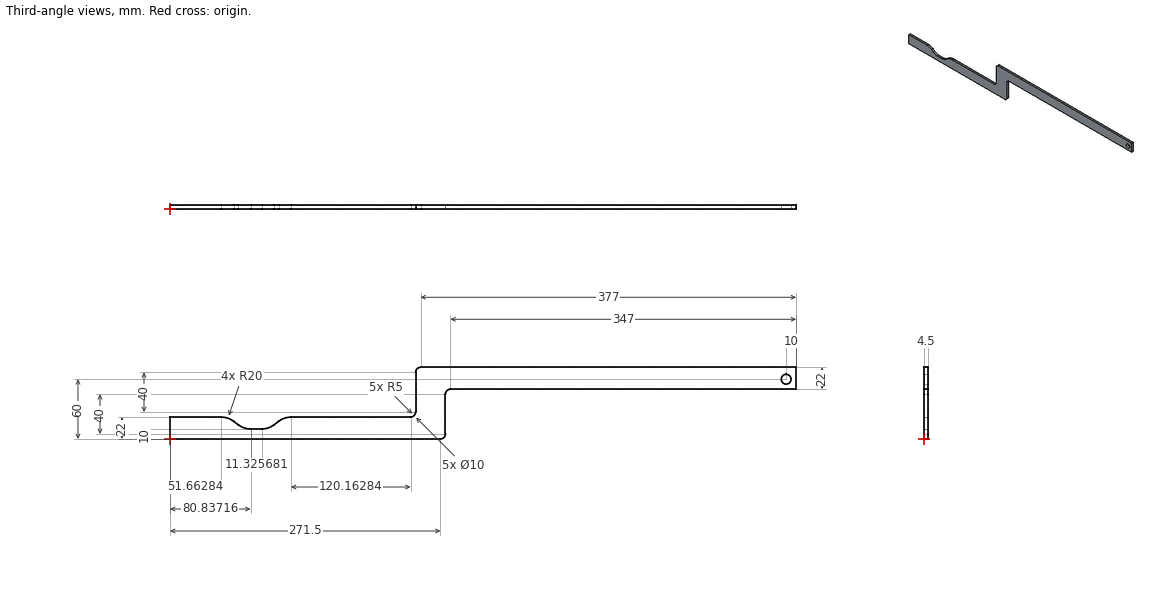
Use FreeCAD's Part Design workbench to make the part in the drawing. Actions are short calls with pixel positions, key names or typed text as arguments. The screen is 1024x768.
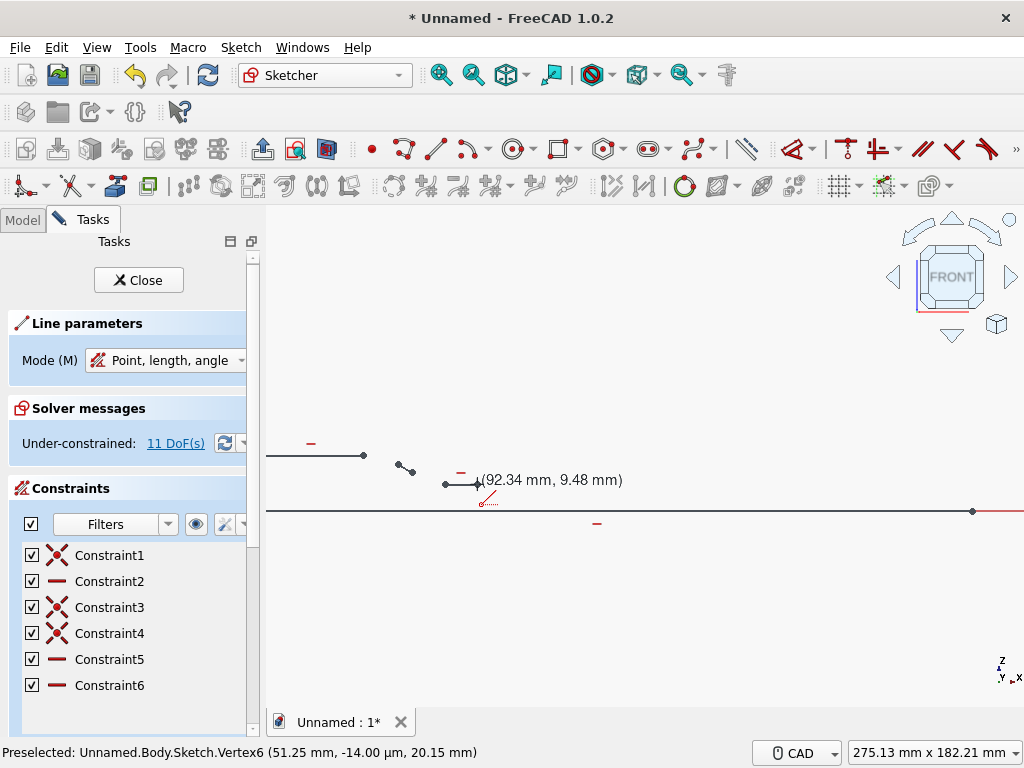
click(510, 472)
click(523, 462)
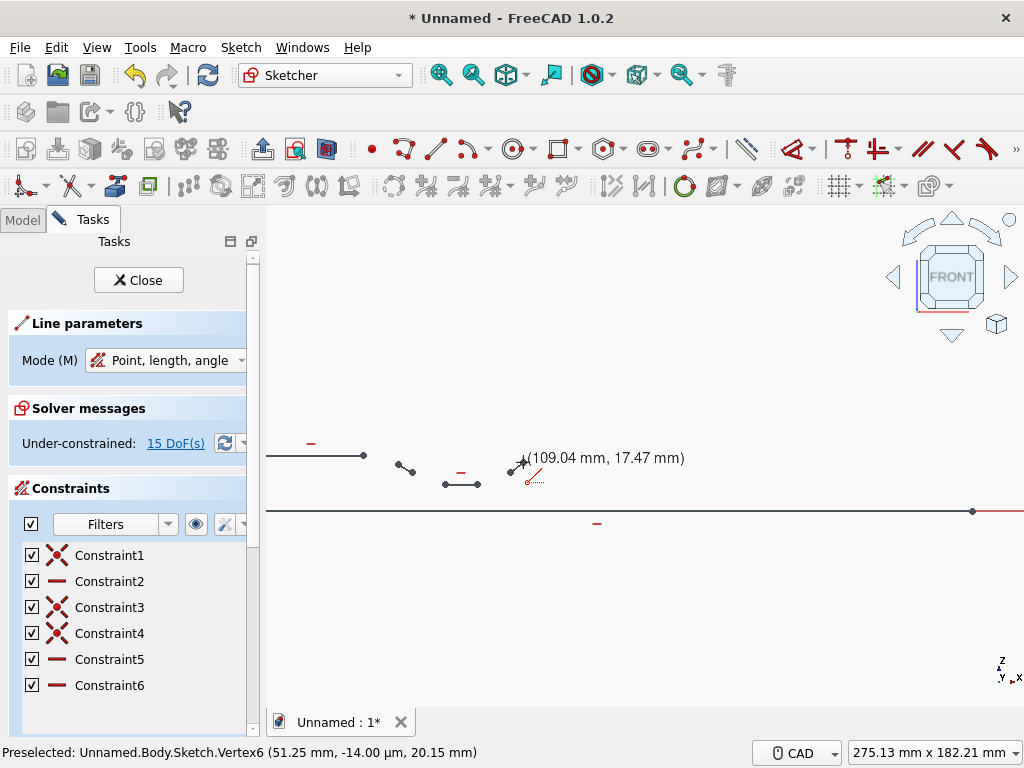
click(557, 451)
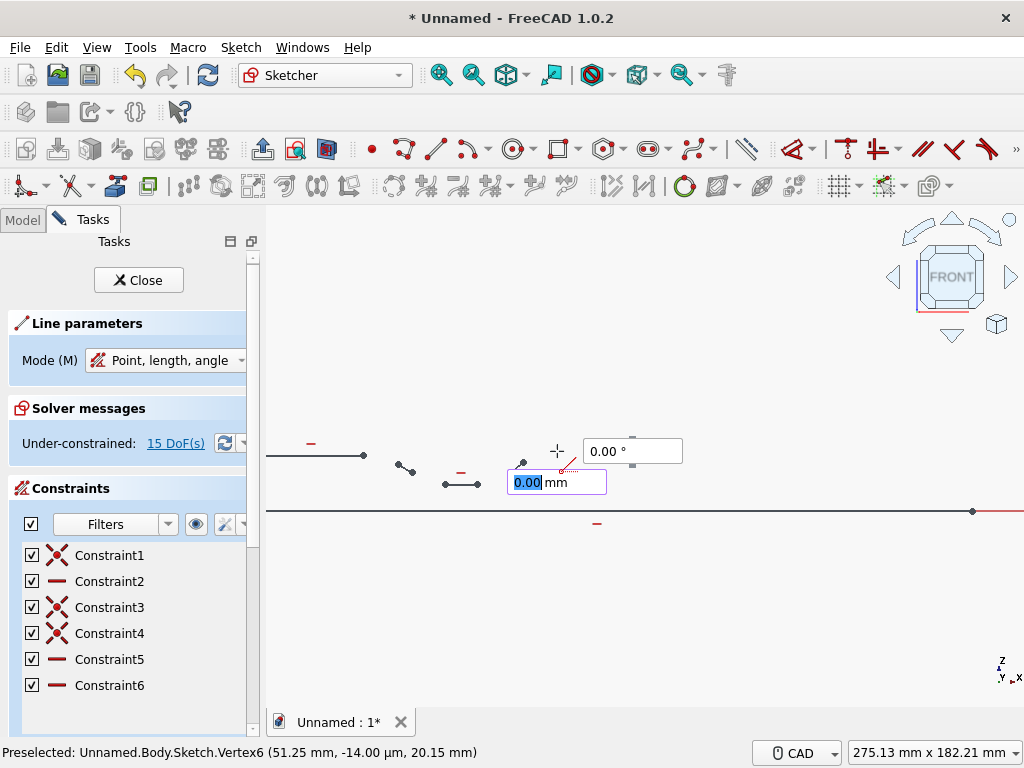
scroll(409, 470, down, 7)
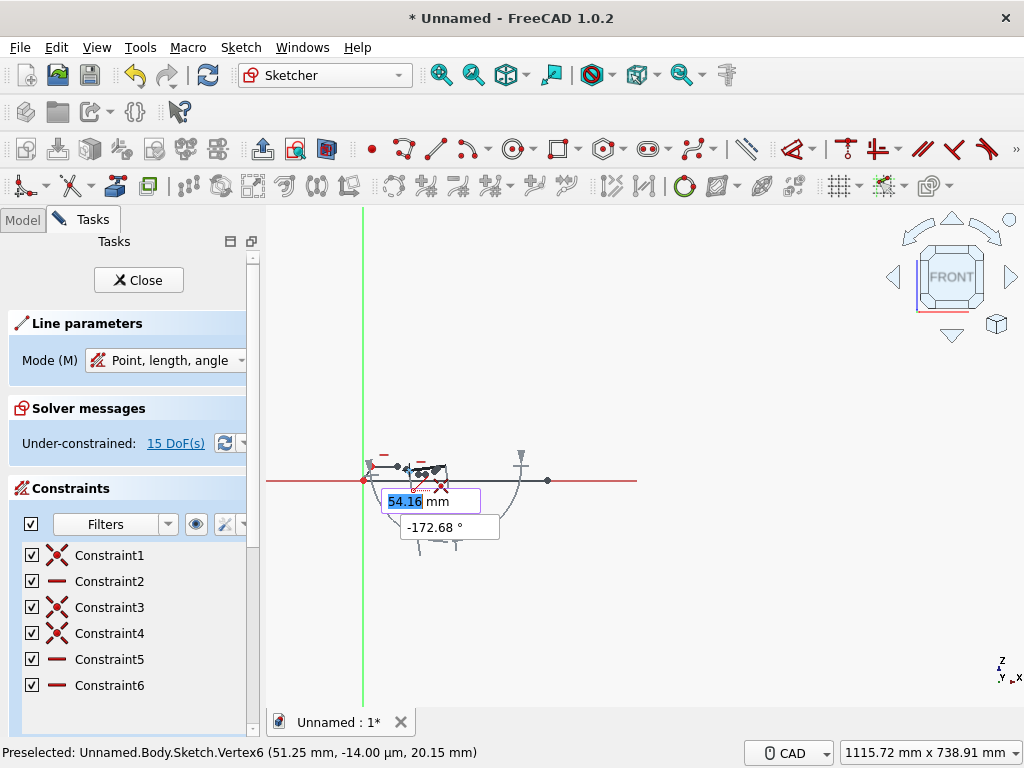
click(527, 466)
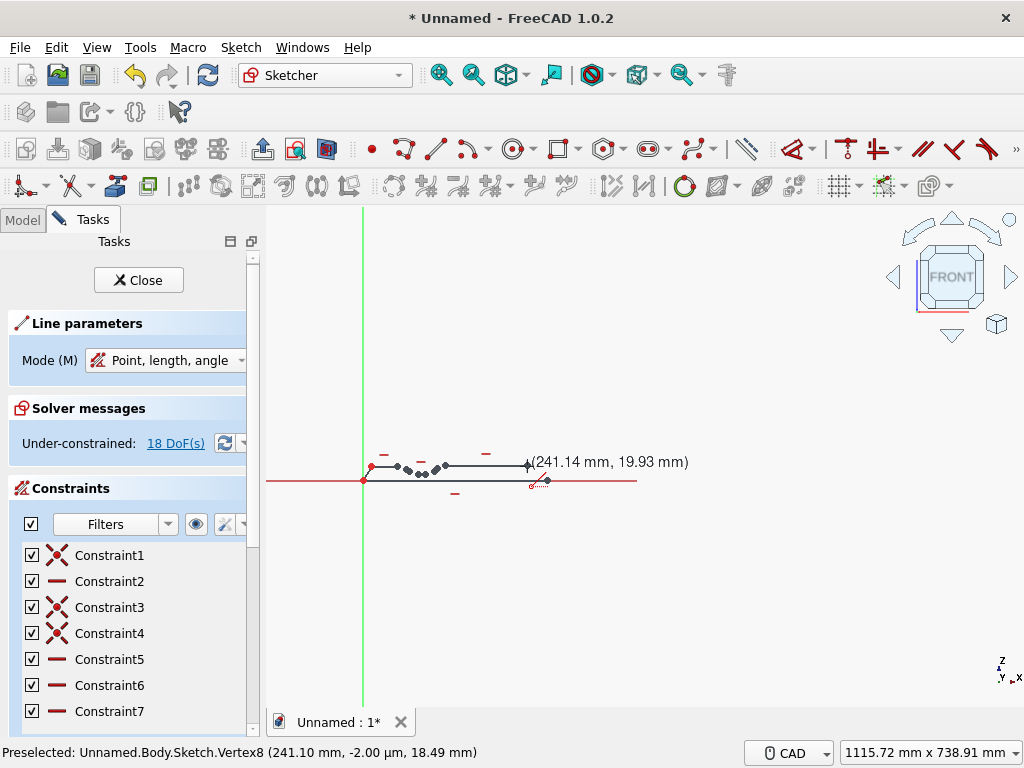
scroll(531, 462, up, 6)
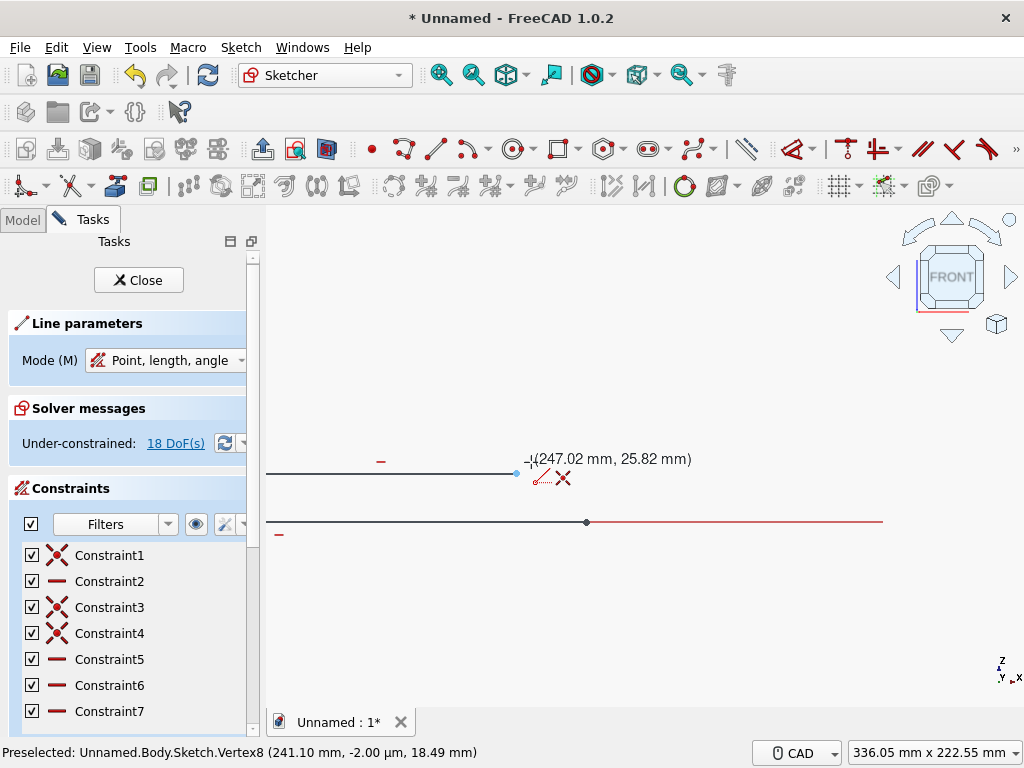
click(529, 461)
click(529, 371)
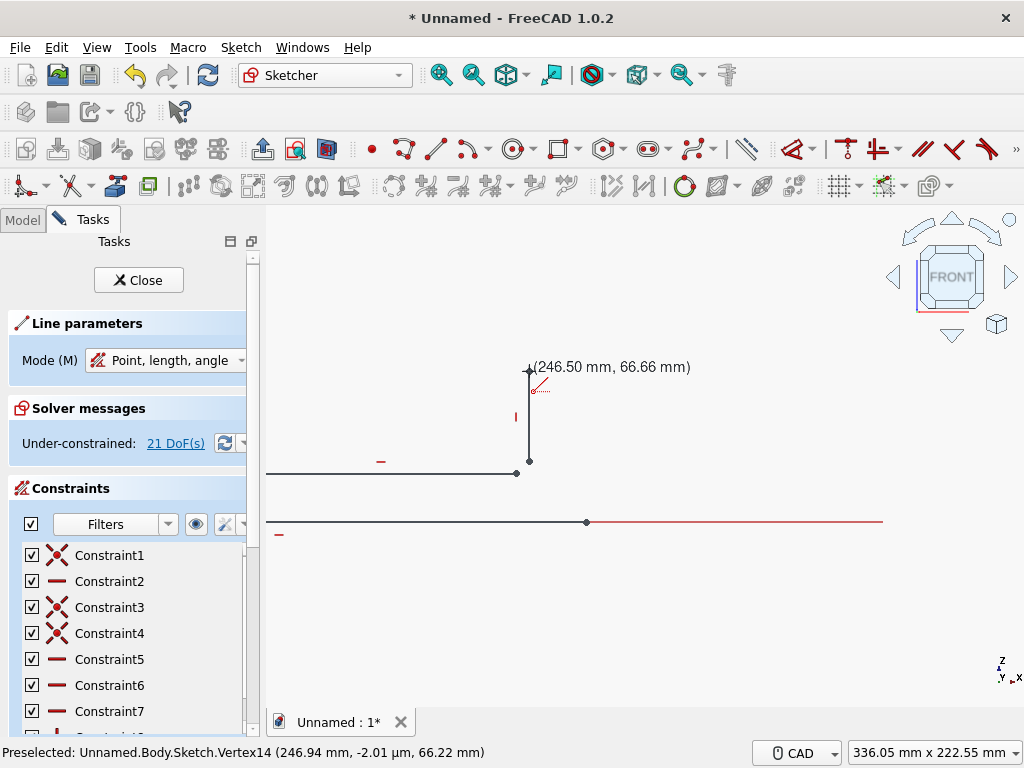
key(g)
key(m)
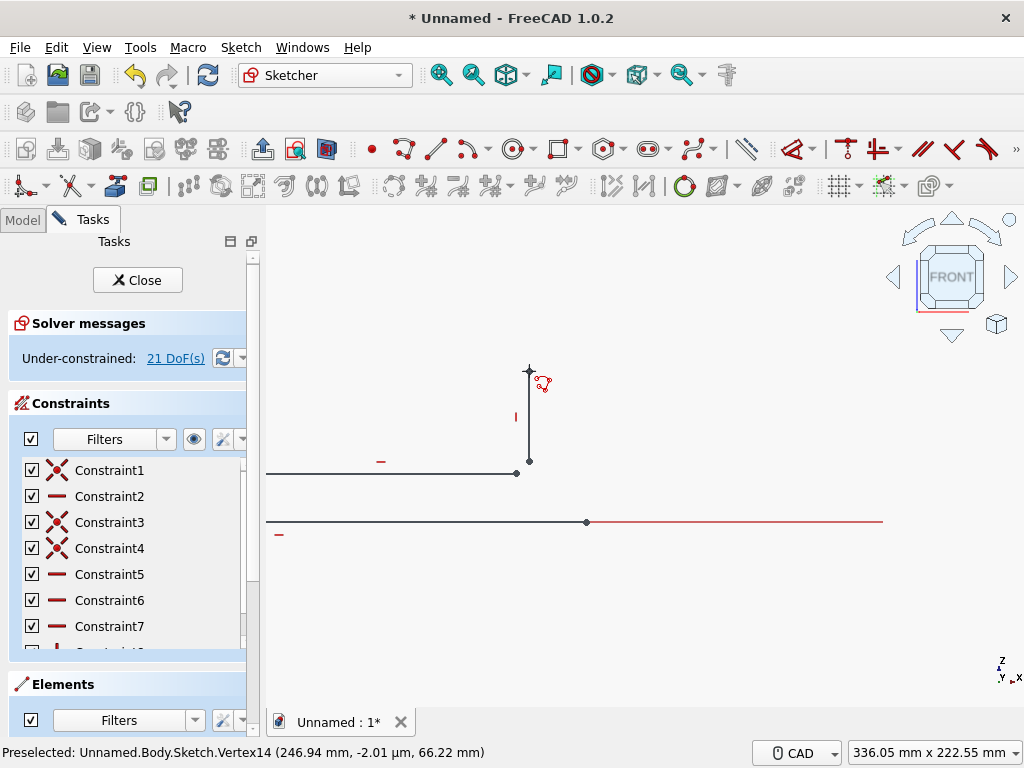
click(540, 360)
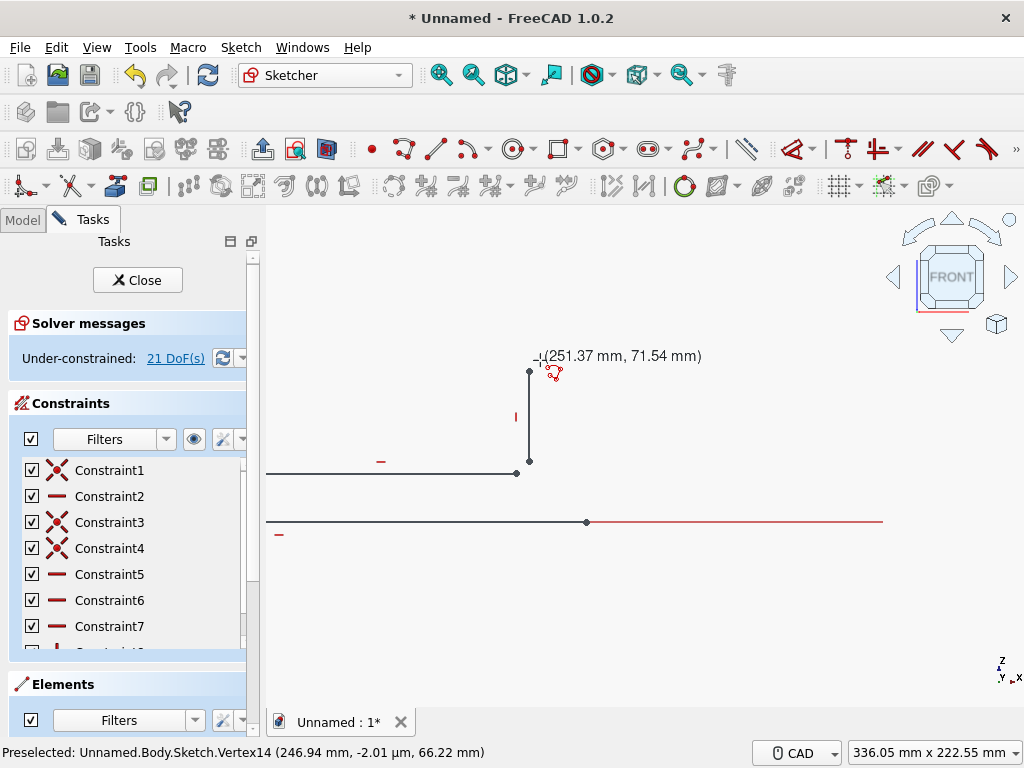
scroll(531, 462, down, 6)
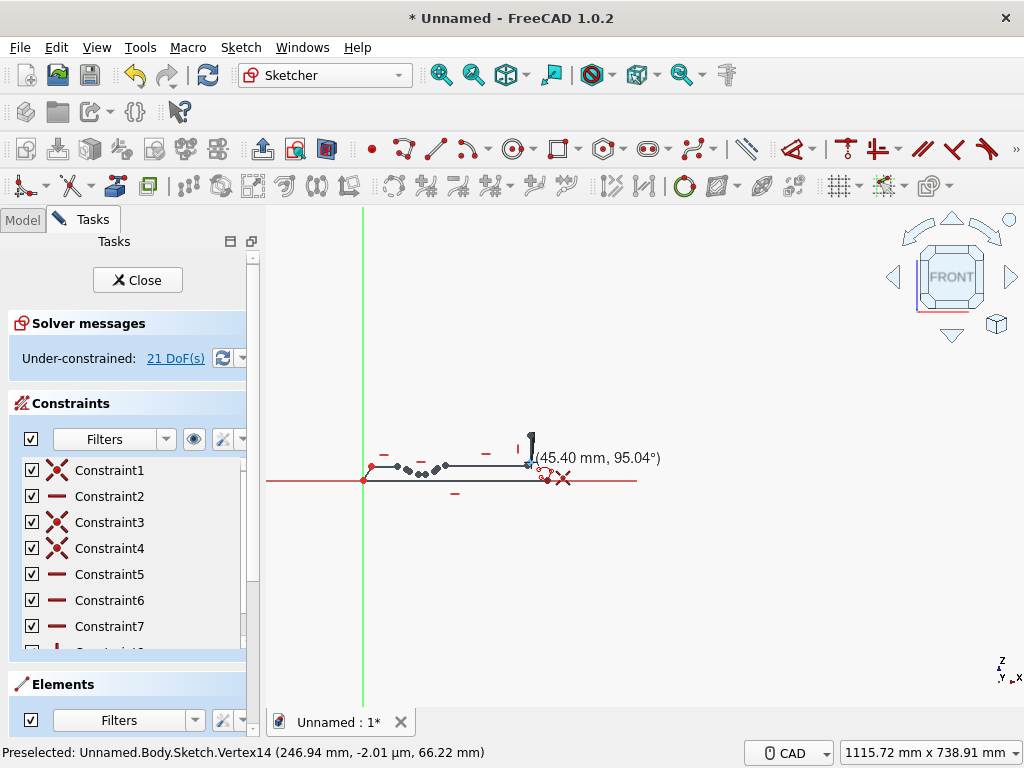
click(790, 432)
click(790, 447)
click(554, 447)
right_click(554, 447)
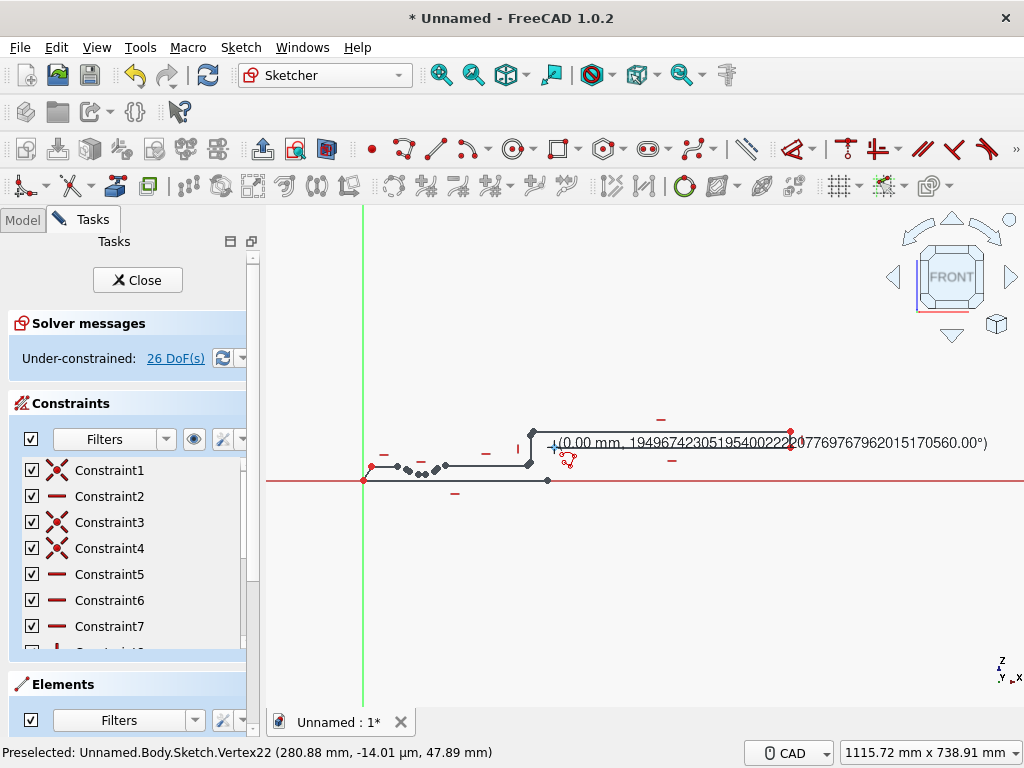
click(436, 150)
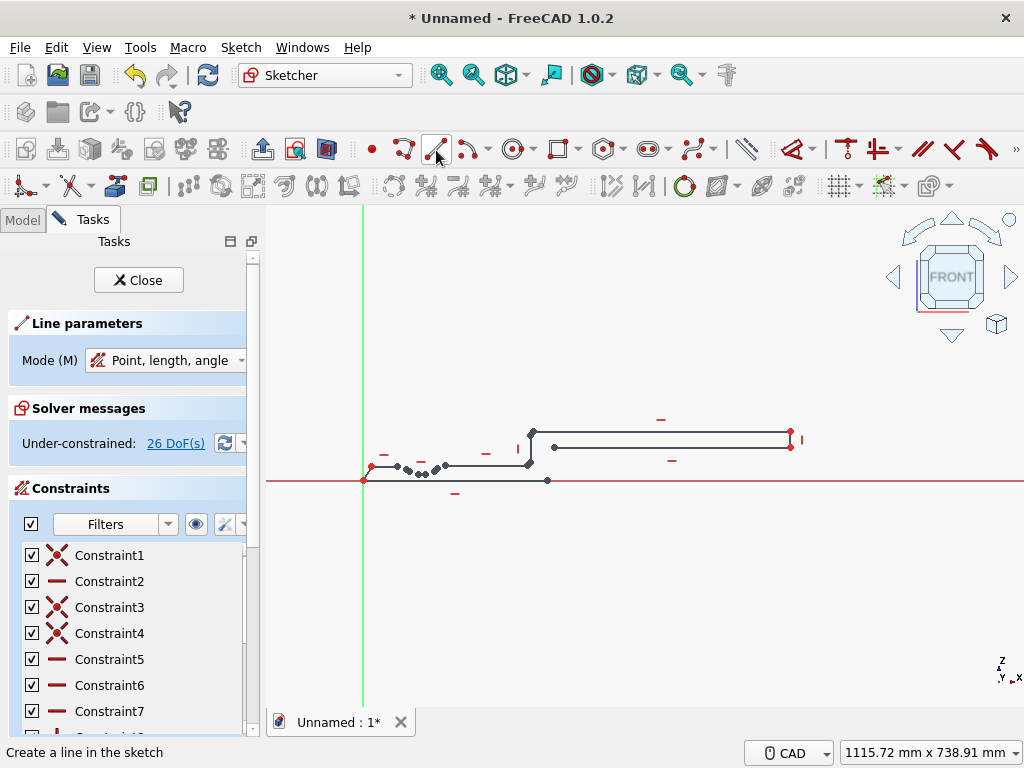
scroll(551, 450, up, 6)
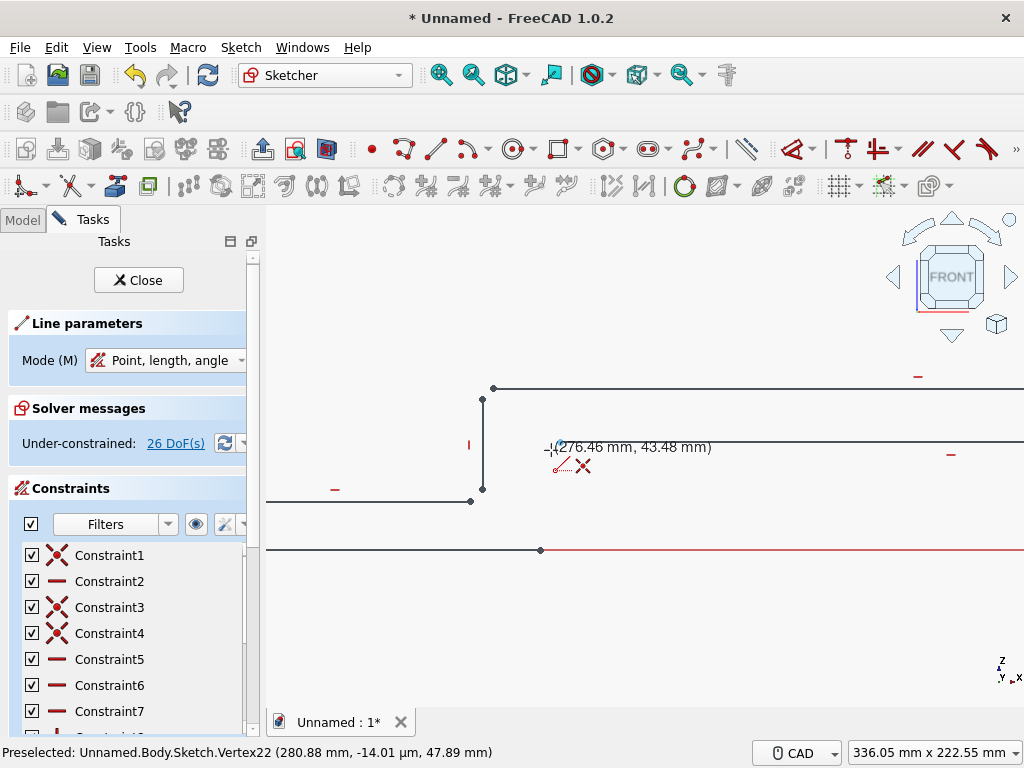
click(550, 449)